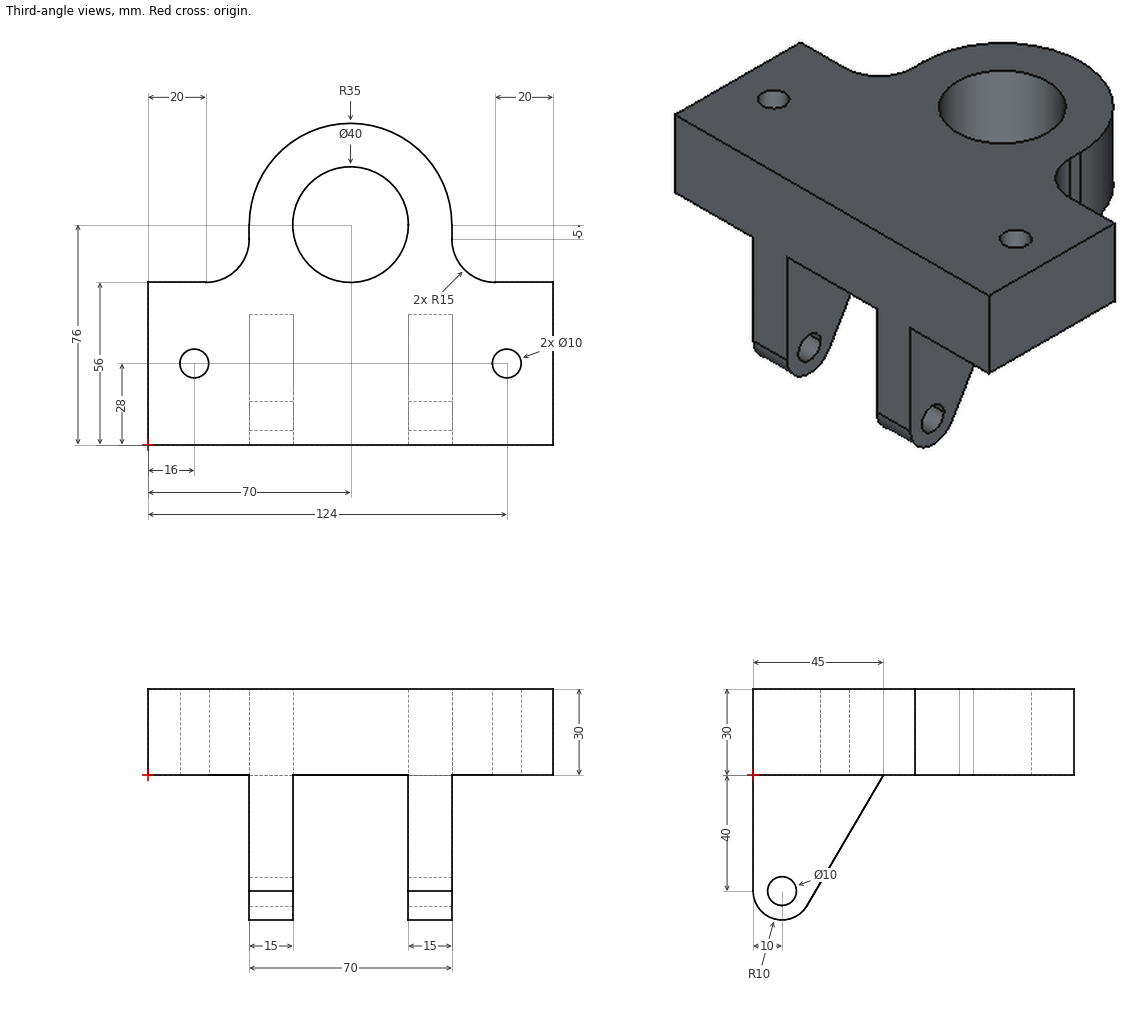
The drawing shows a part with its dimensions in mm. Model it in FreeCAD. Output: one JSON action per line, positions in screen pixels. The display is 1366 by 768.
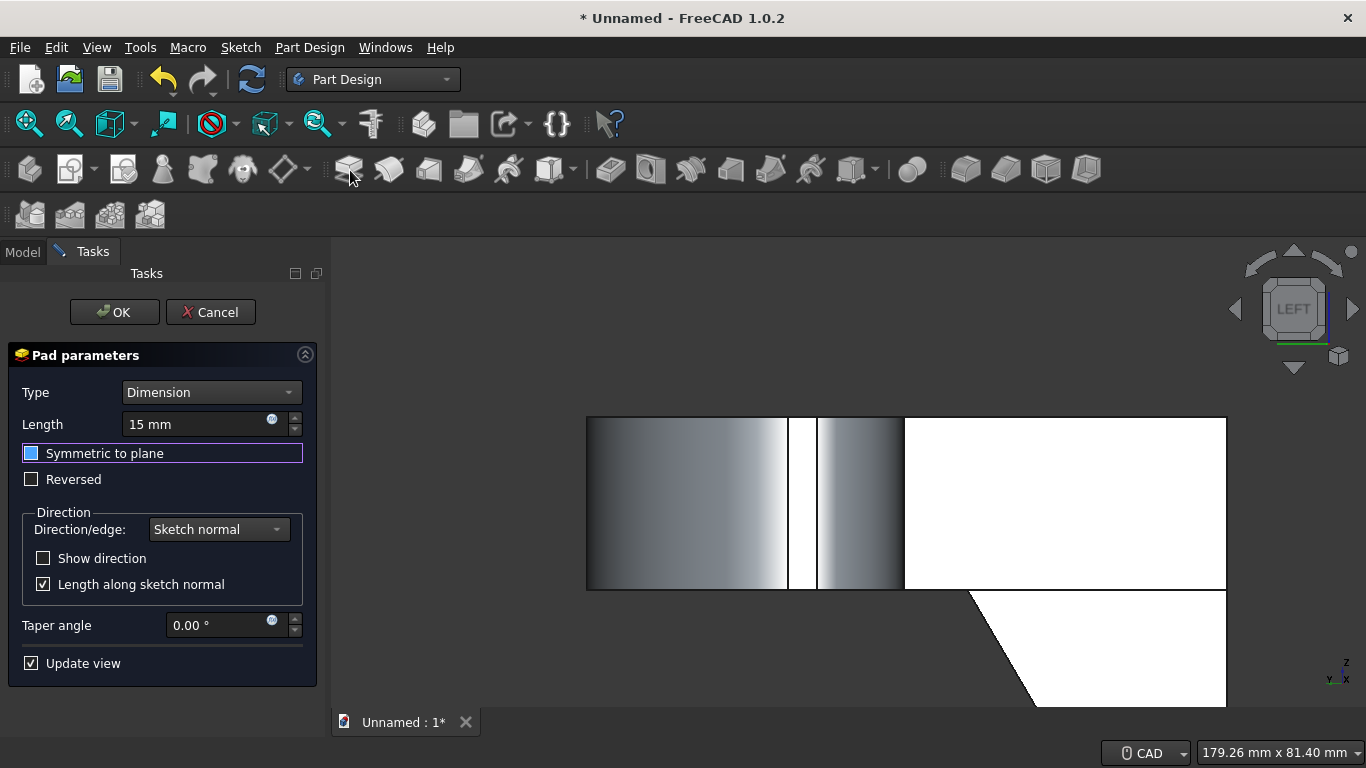
{"action": "left_click", "coordinate": [30, 479]}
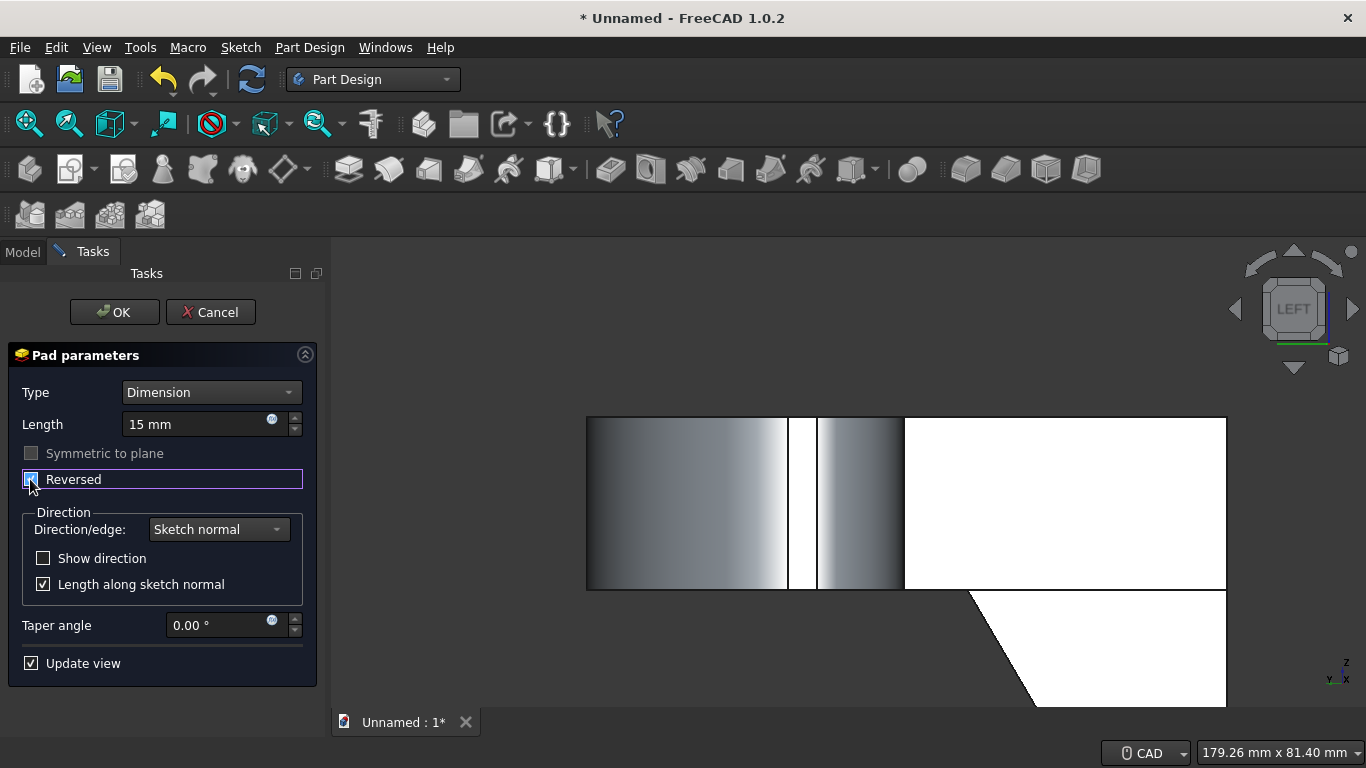
{"action": "left_click", "coordinate": [115, 312]}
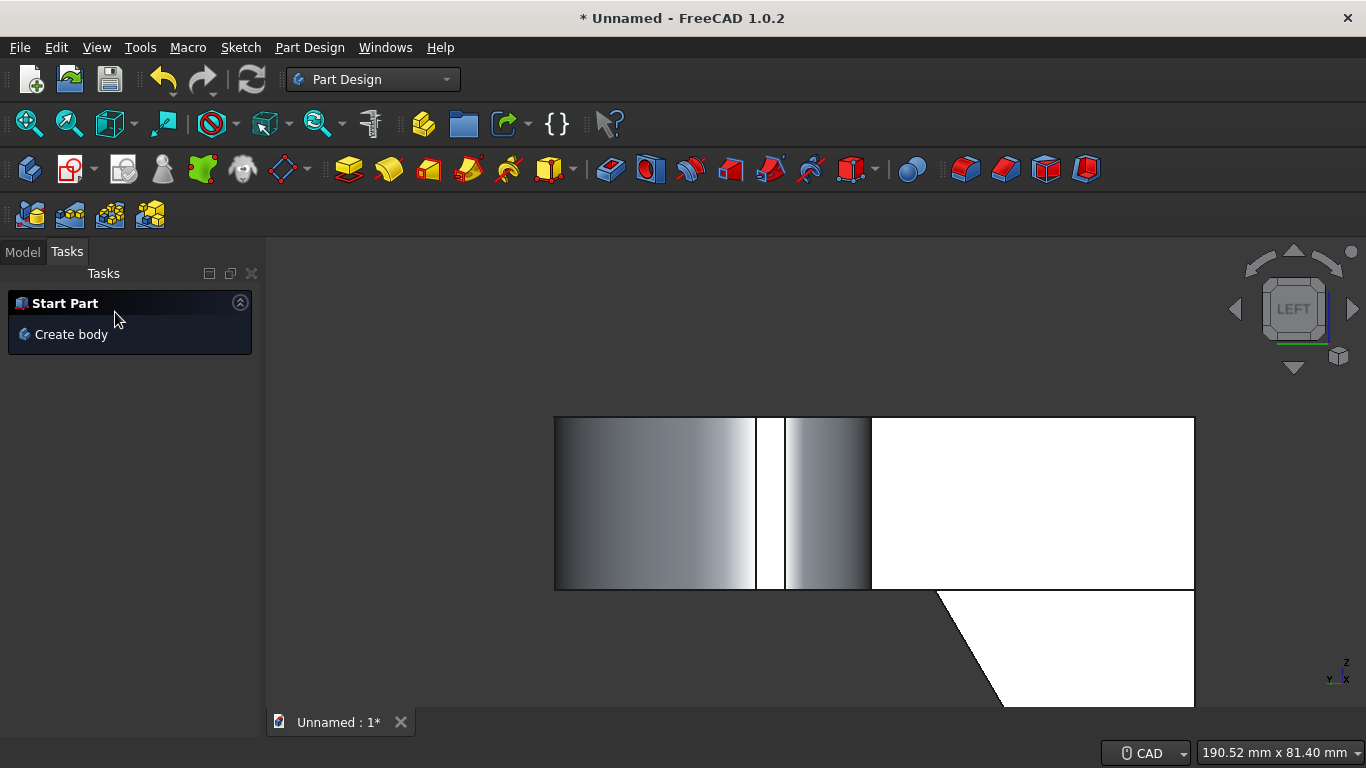
{"action": "left_click", "coordinate": [30, 124]}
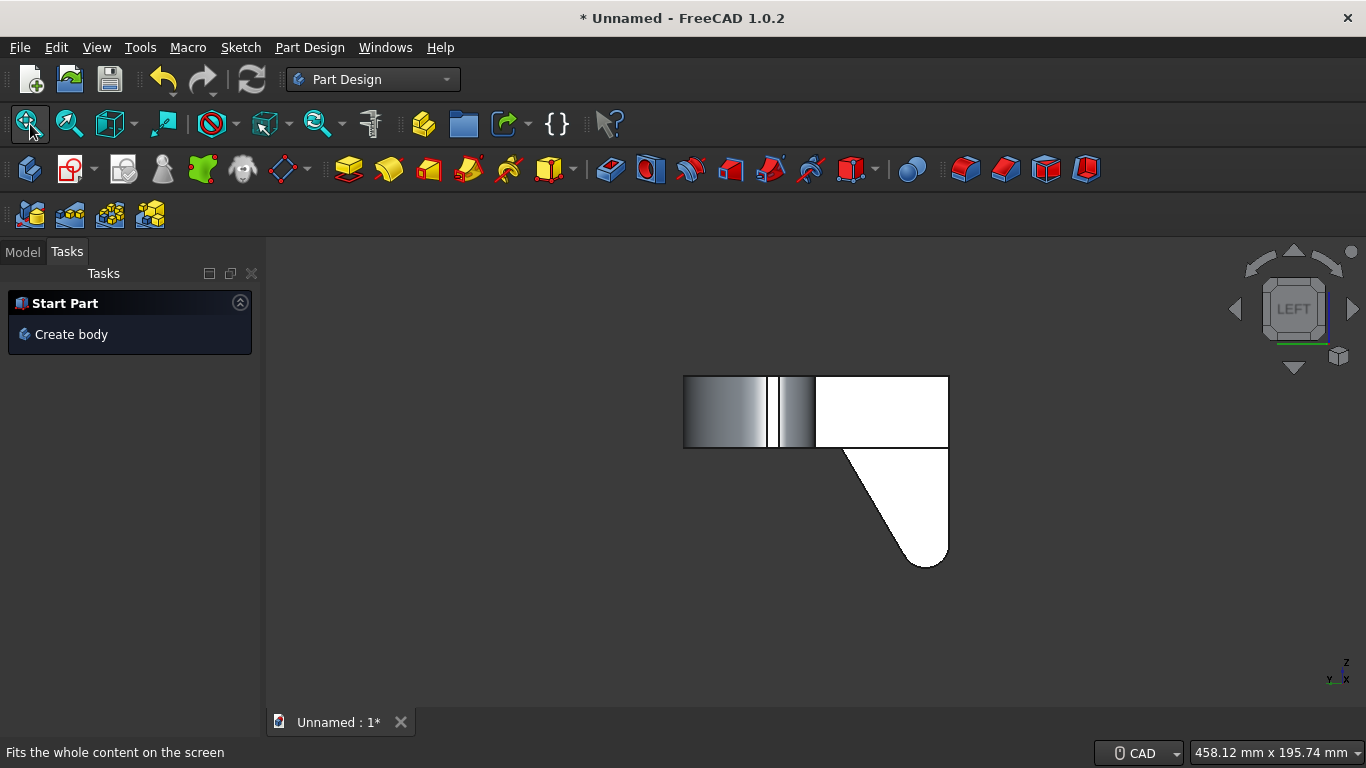
{"action": "left_click", "coordinate": [23, 251]}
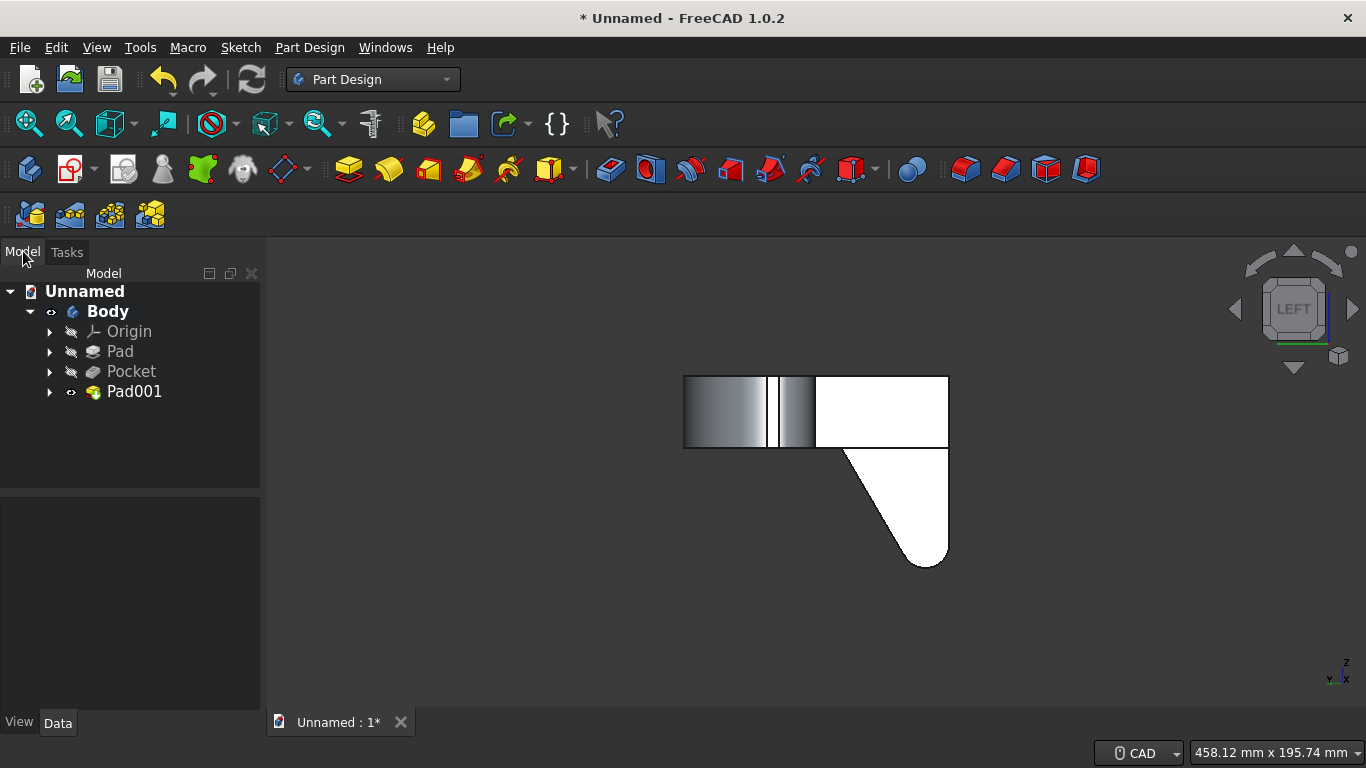
{"action": "left_click", "coordinate": [50, 332]}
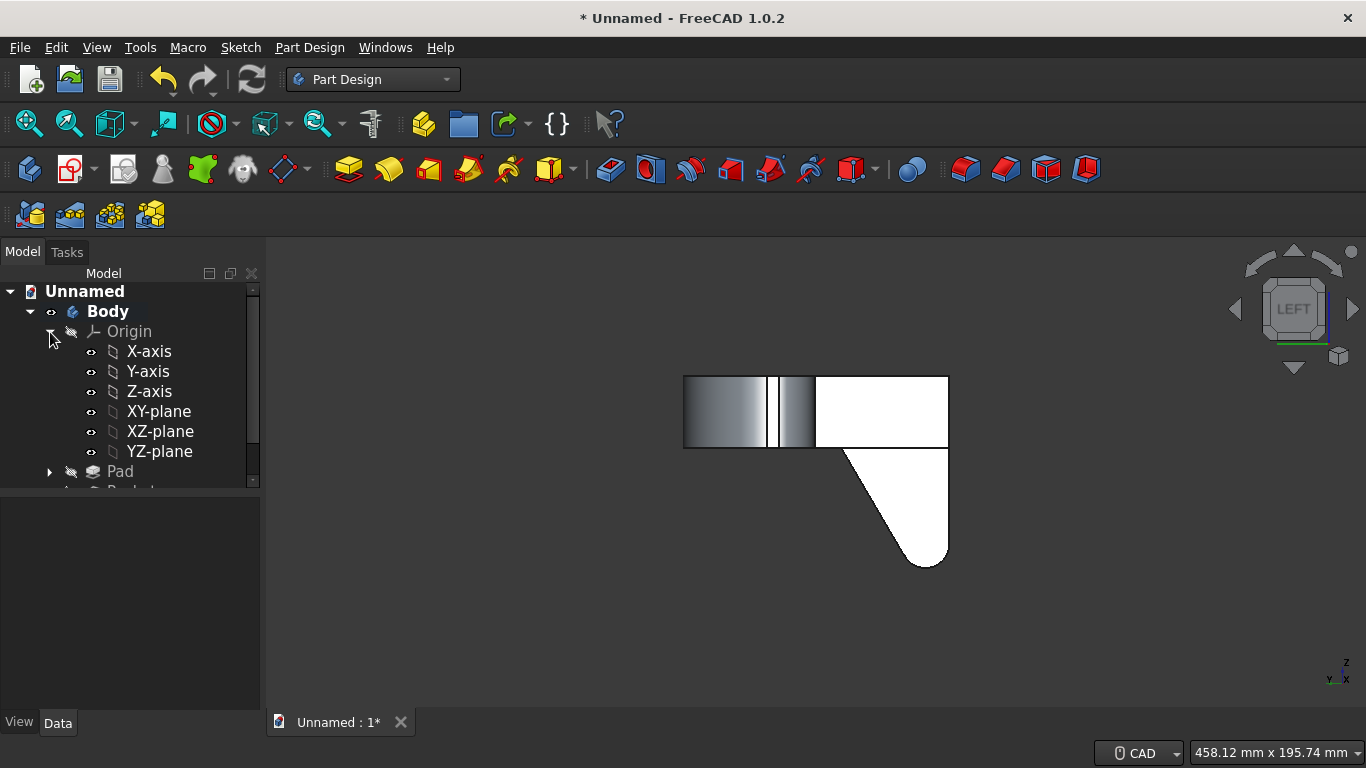
{"action": "left_click", "coordinate": [136, 452]}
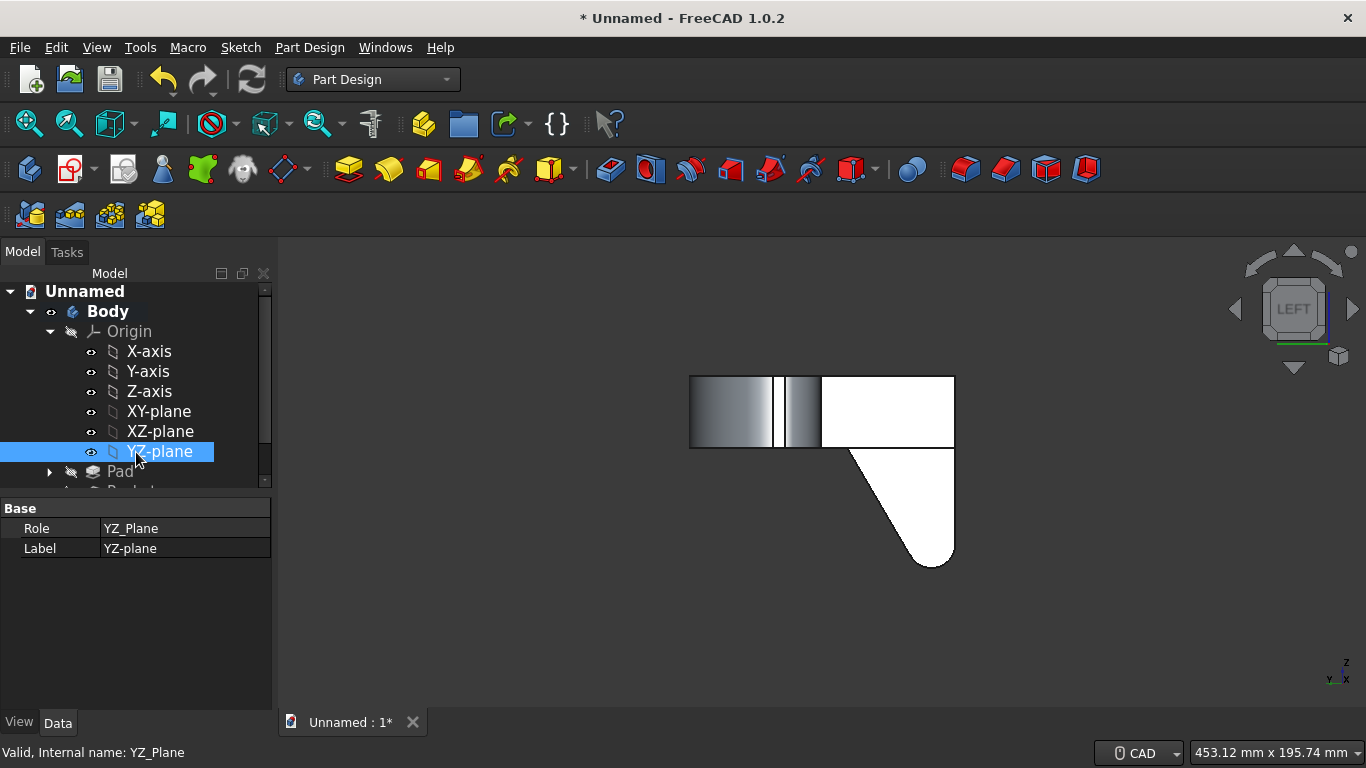
{"action": "left_click", "coordinate": [284, 170]}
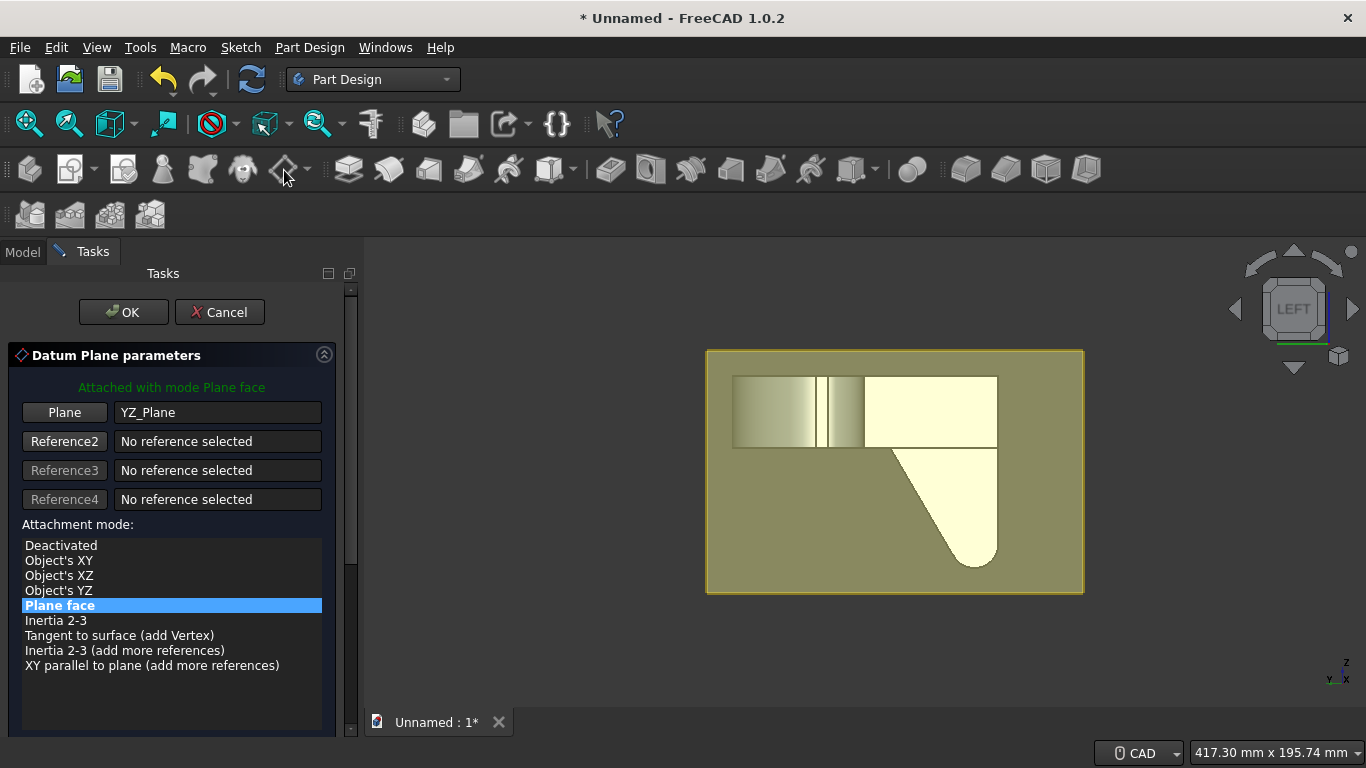
{"action": "scroll", "coordinate": [351, 510], "scroll_direction": "down", "scroll_amount": 3}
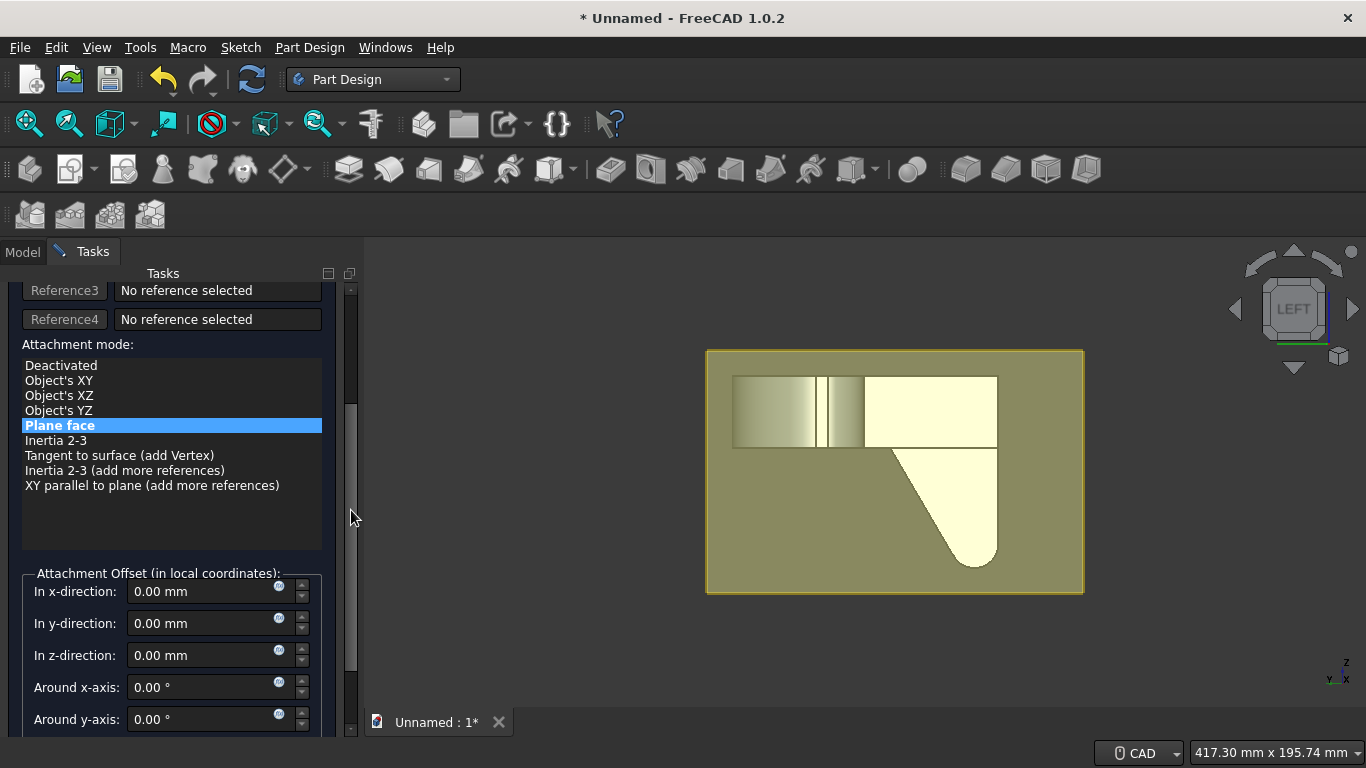
{"action": "triple_click", "coordinate": [210, 655]}